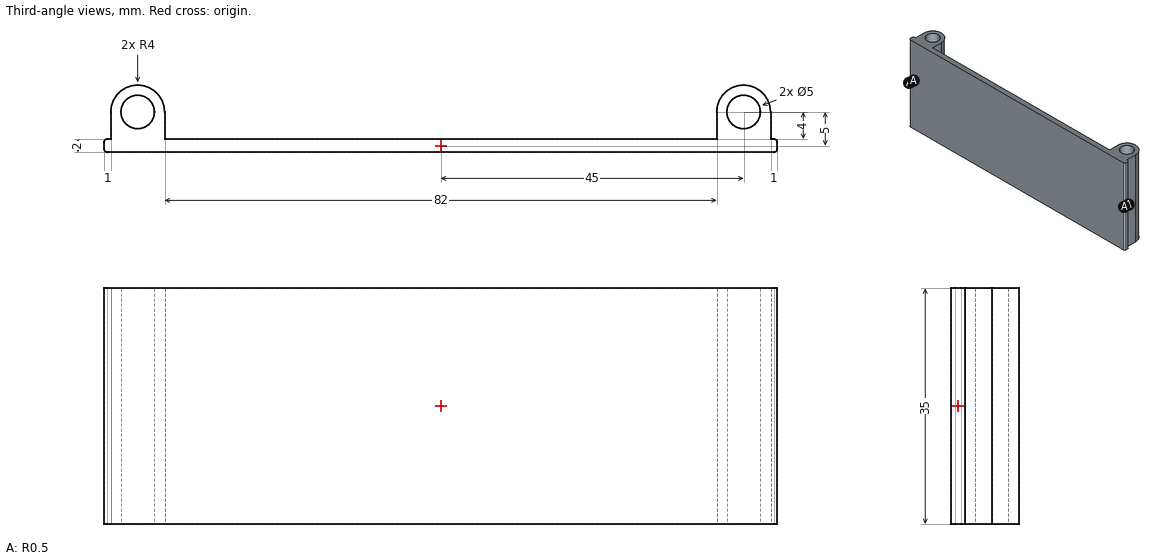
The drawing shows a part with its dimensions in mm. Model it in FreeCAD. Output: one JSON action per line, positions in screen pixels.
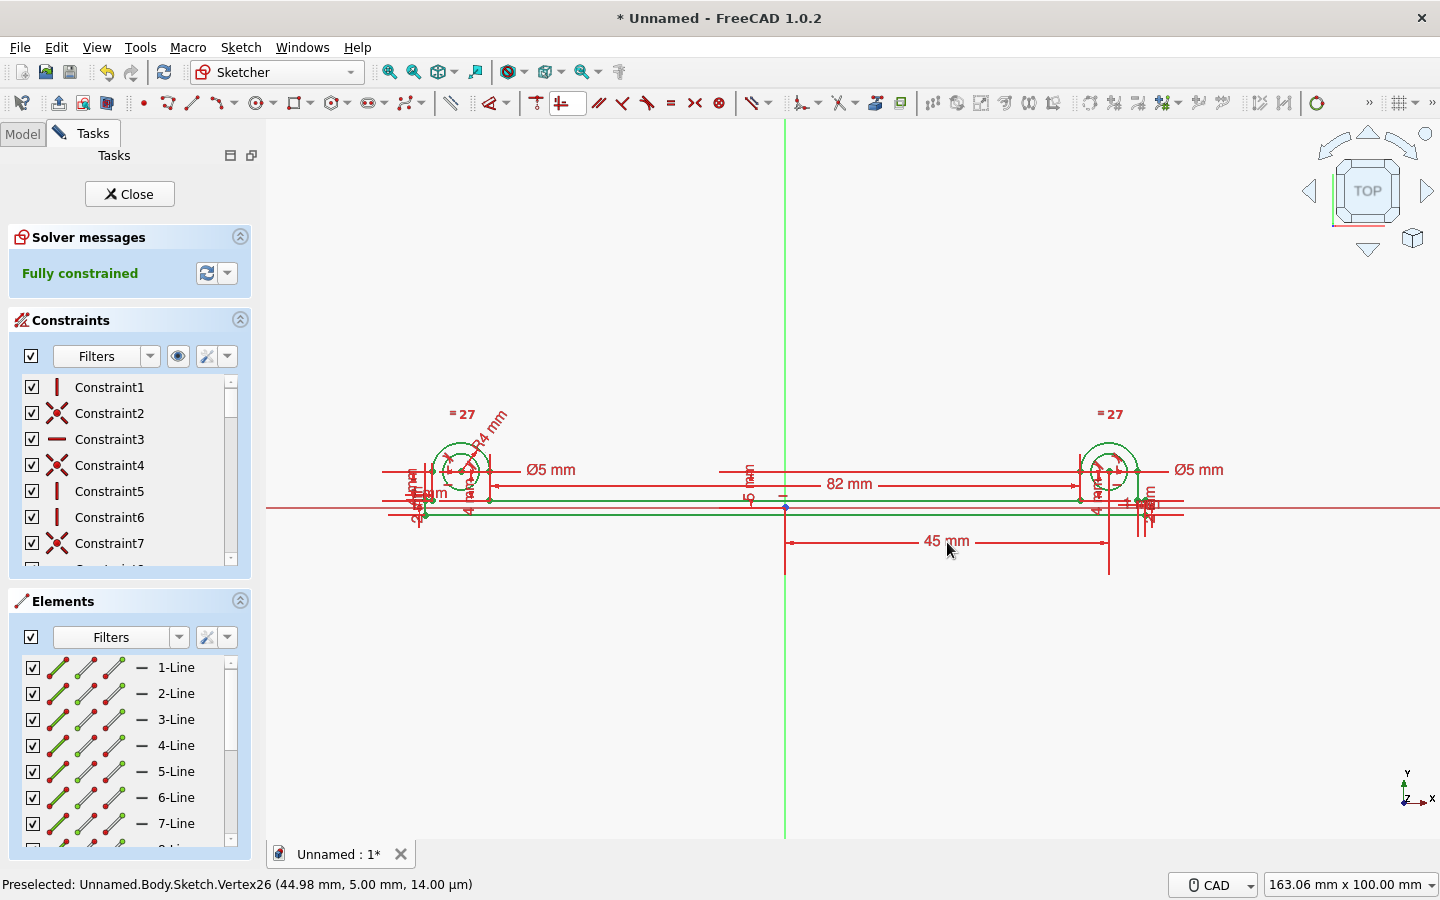
{"action": "left_click", "coordinate": [130, 194]}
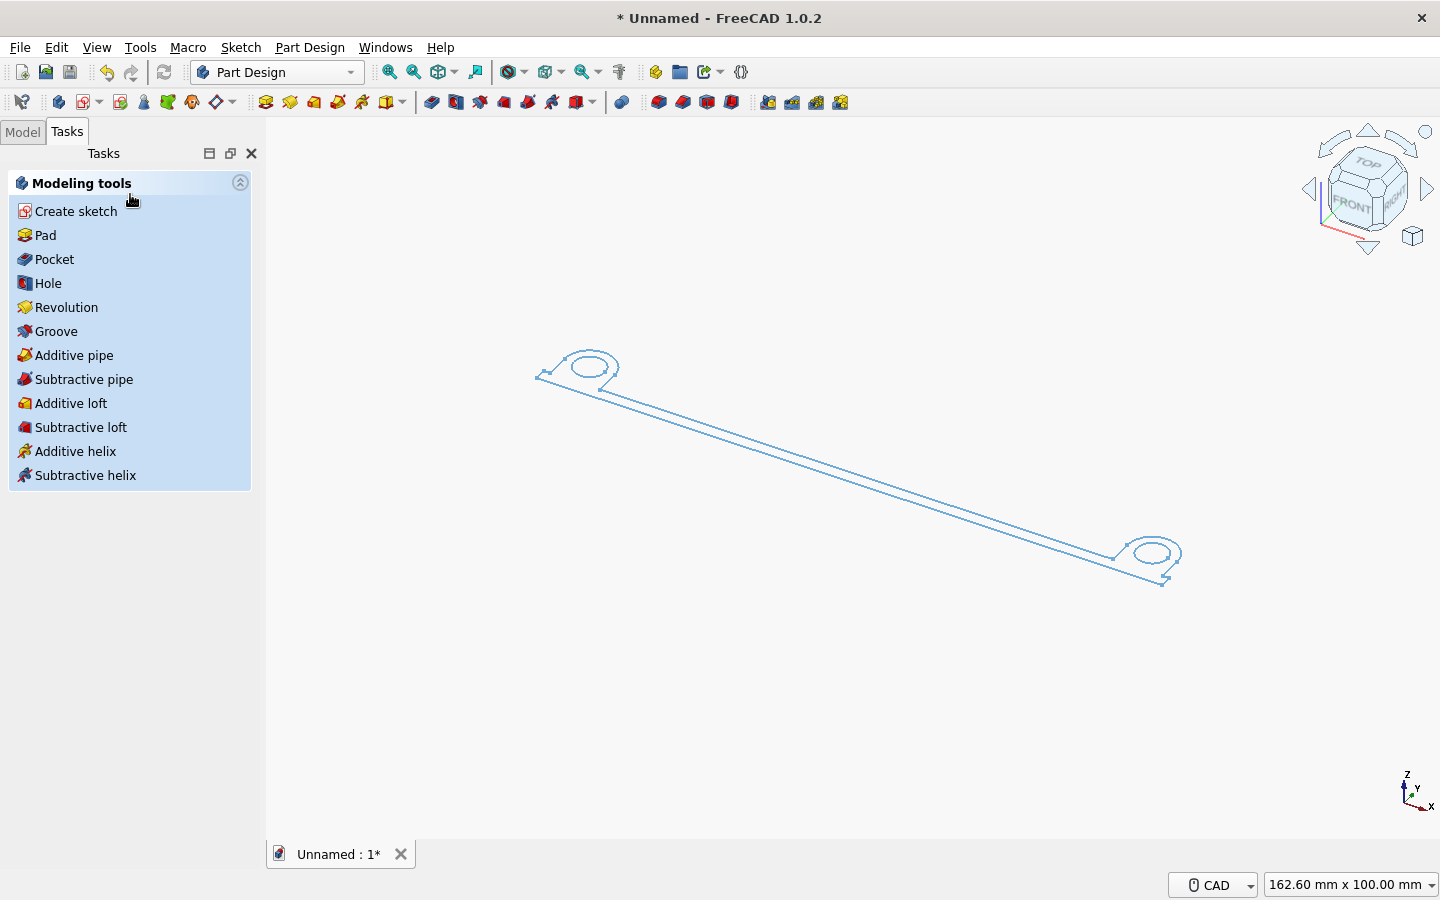
{"action": "left_click", "coordinate": [266, 102]}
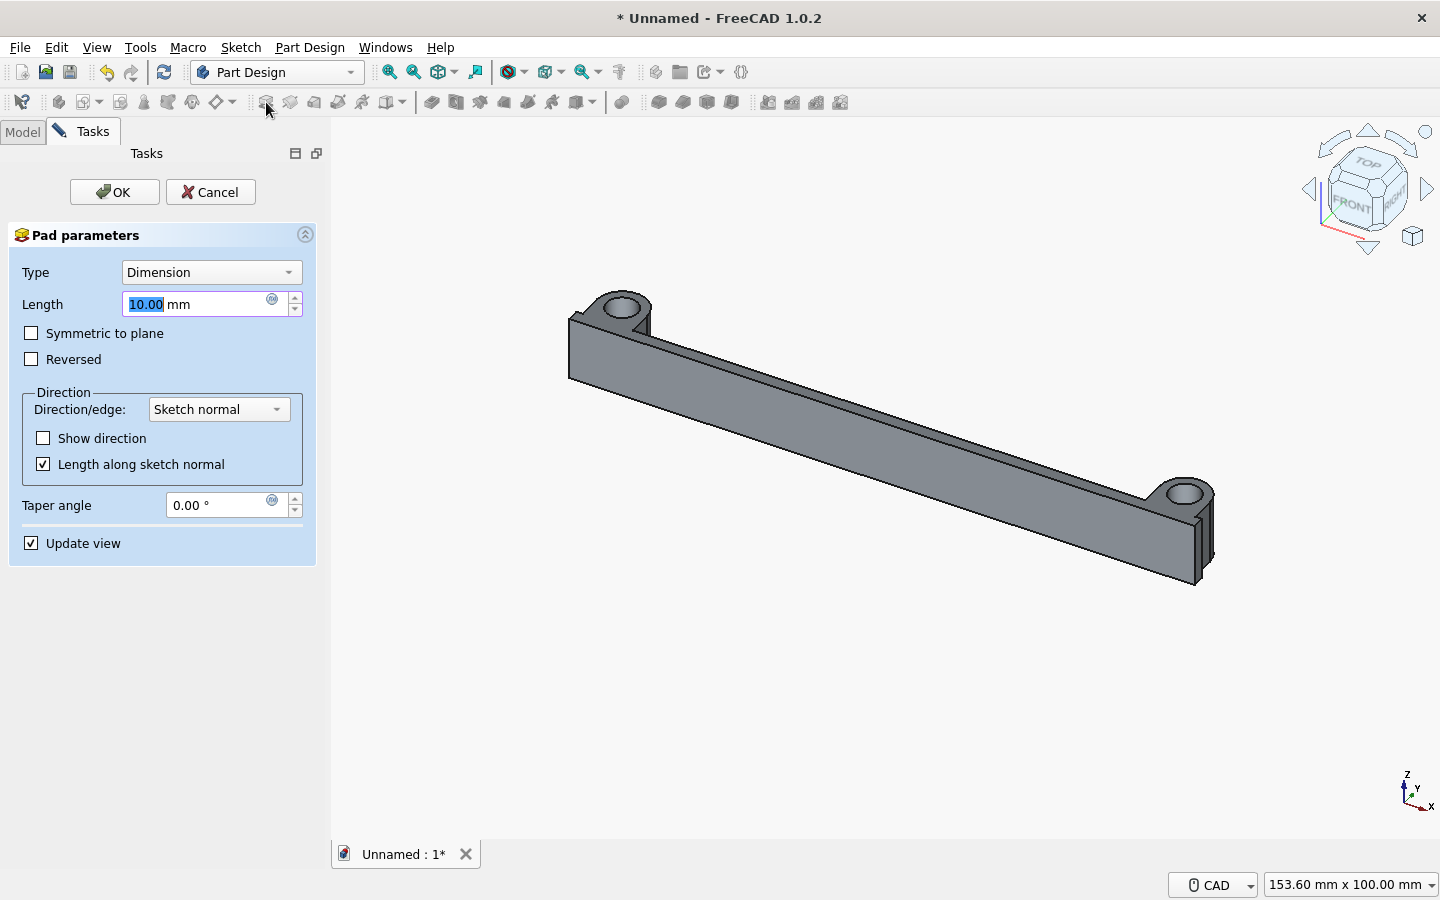
{"action": "type", "text": "35"}
{"action": "key", "text": "Tab"}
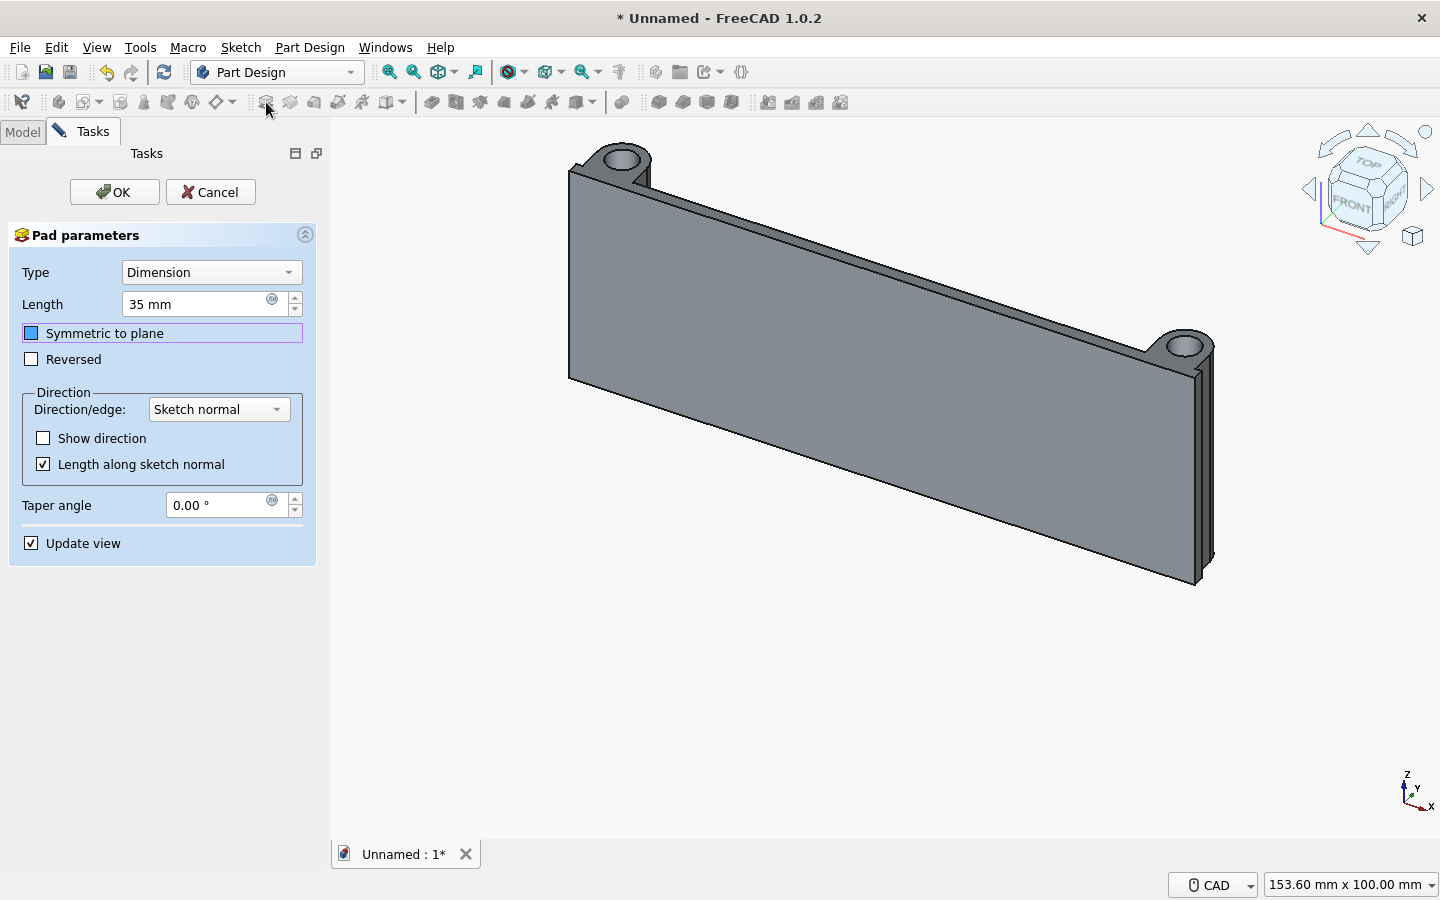
{"action": "left_click", "coordinate": [30, 333]}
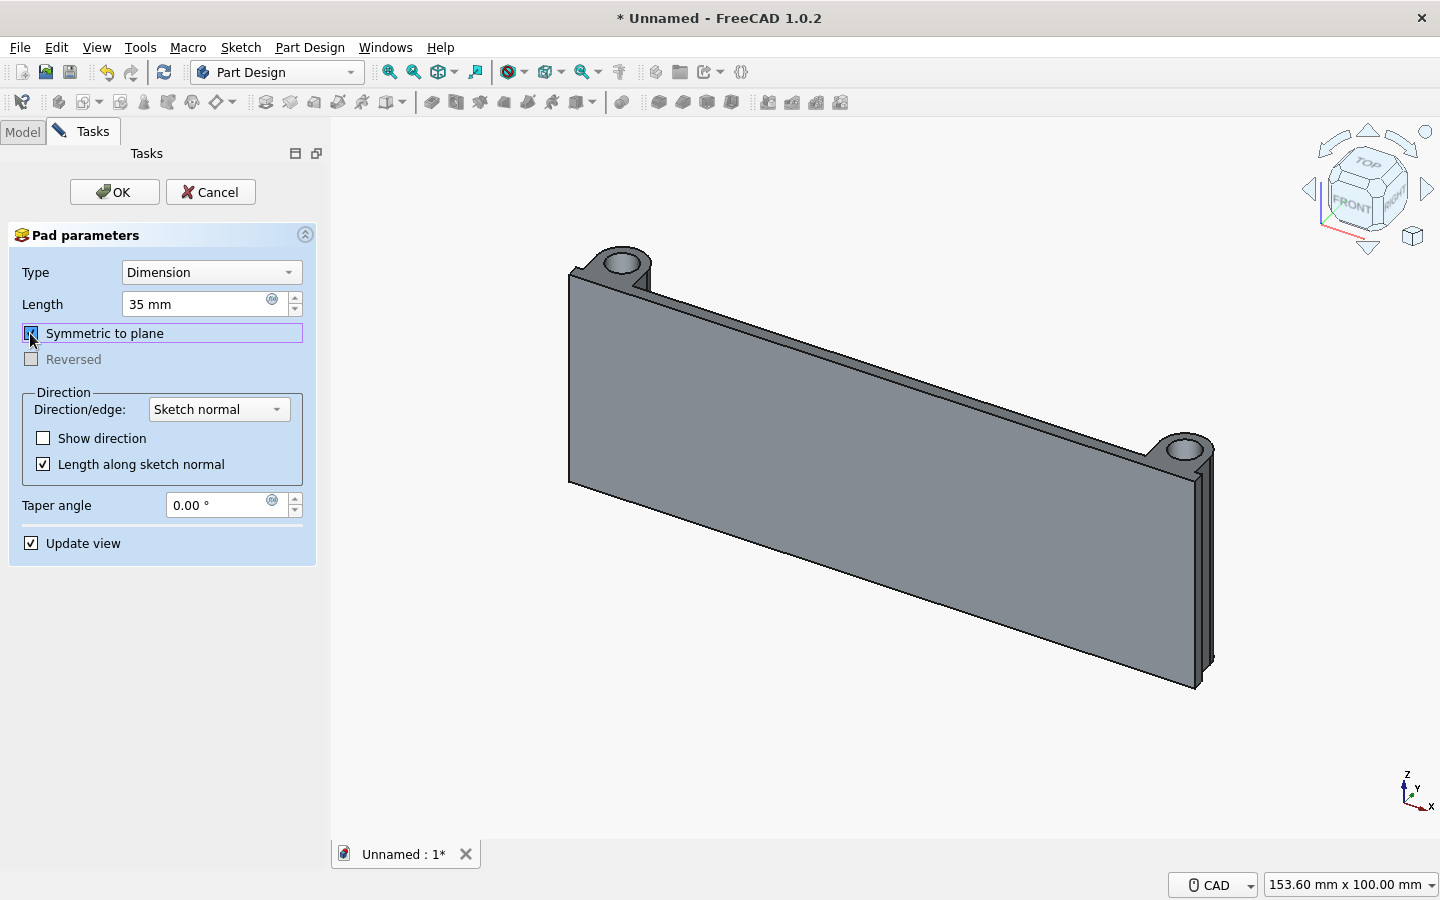
{"action": "left_click", "coordinate": [115, 192]}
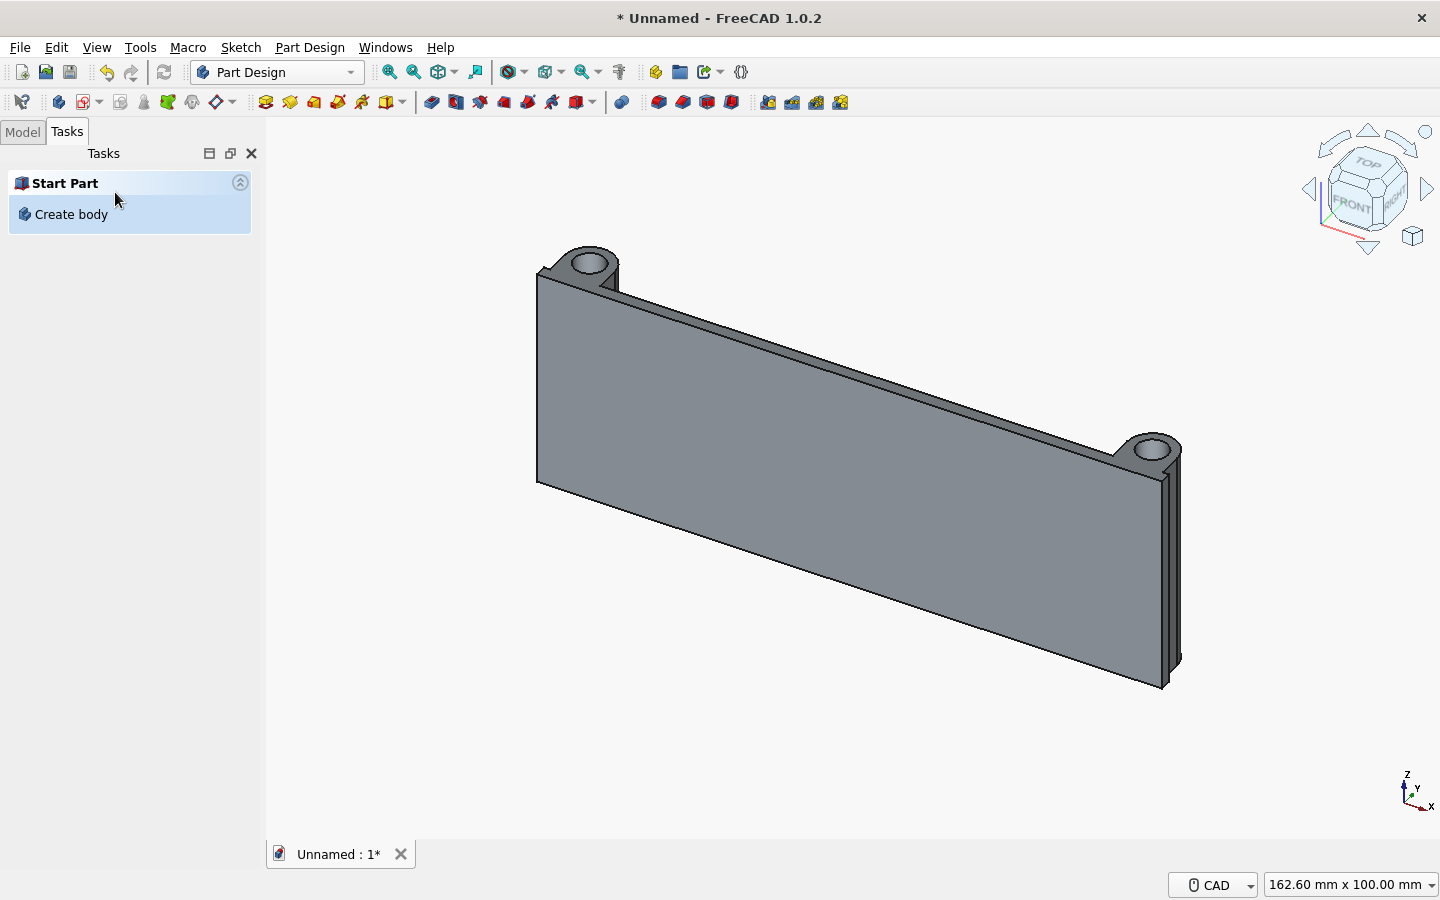
{"action": "left_click", "coordinate": [1162, 584]}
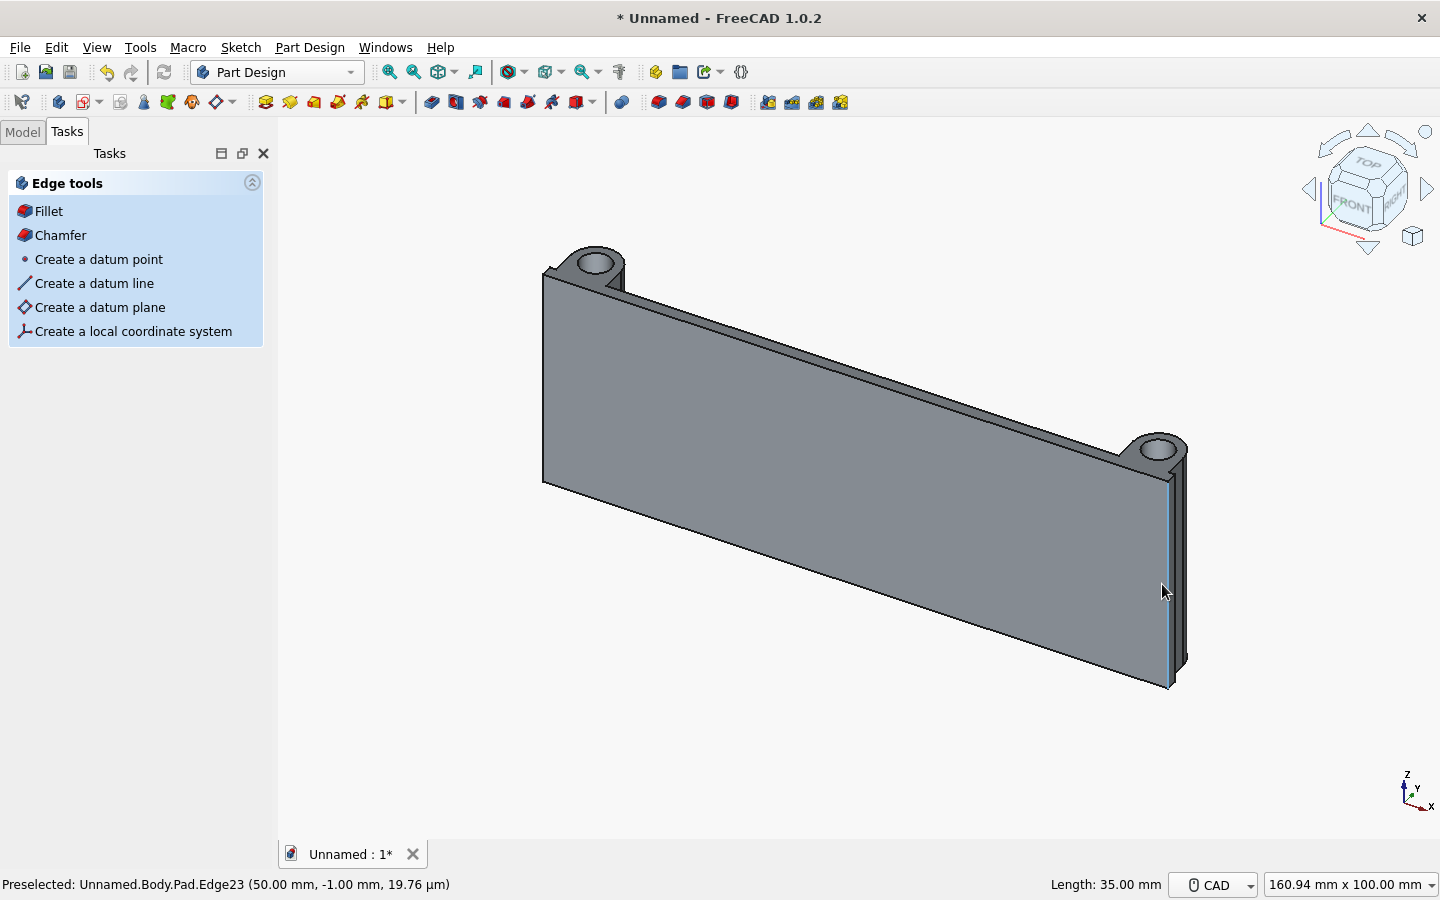
{"action": "key", "text": "0"}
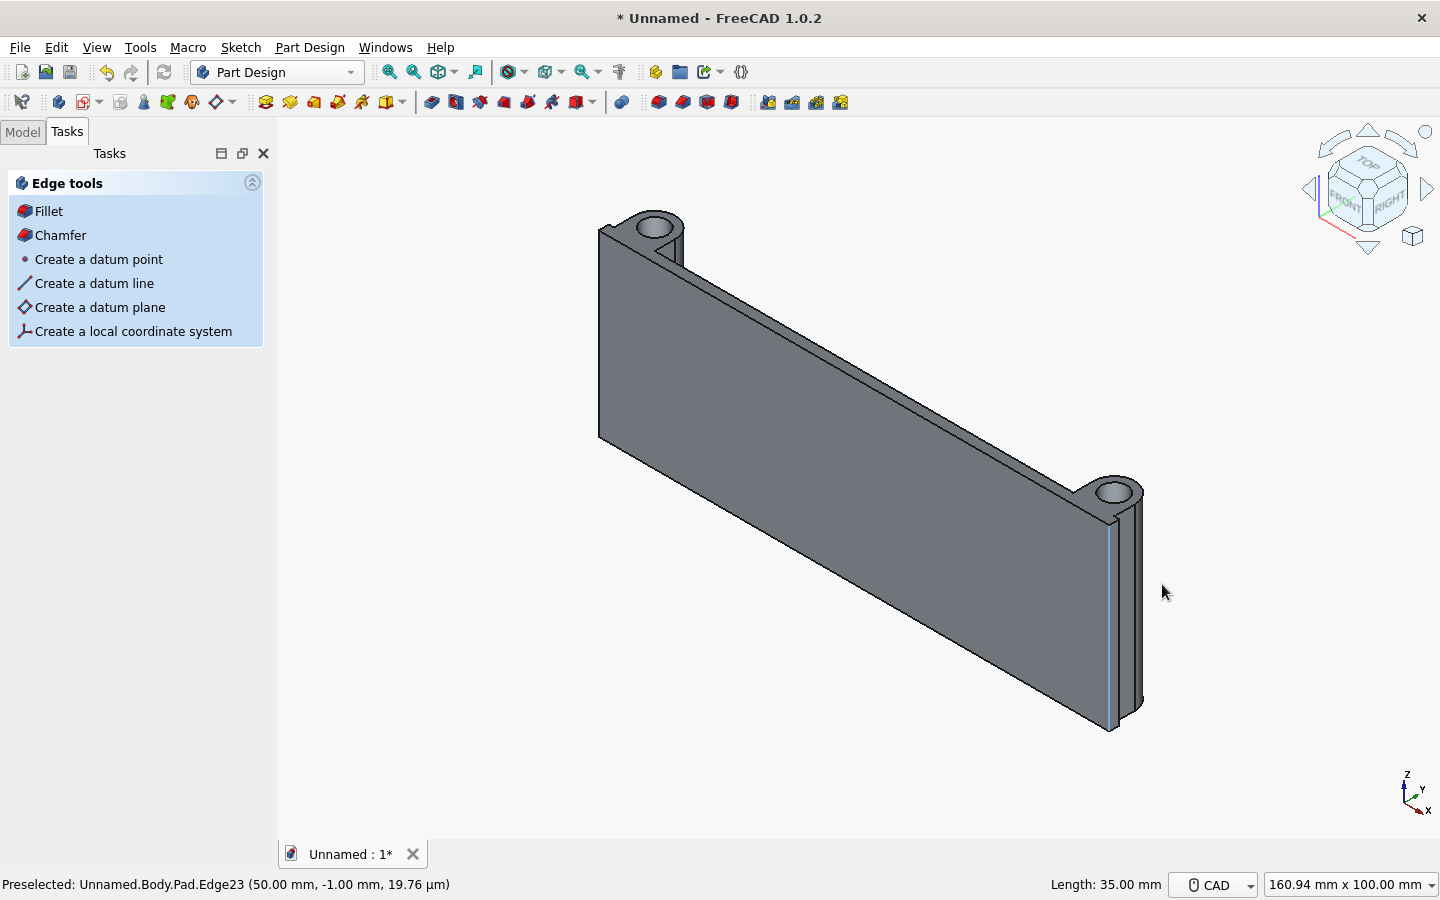
{"action": "key", "text": "2"}